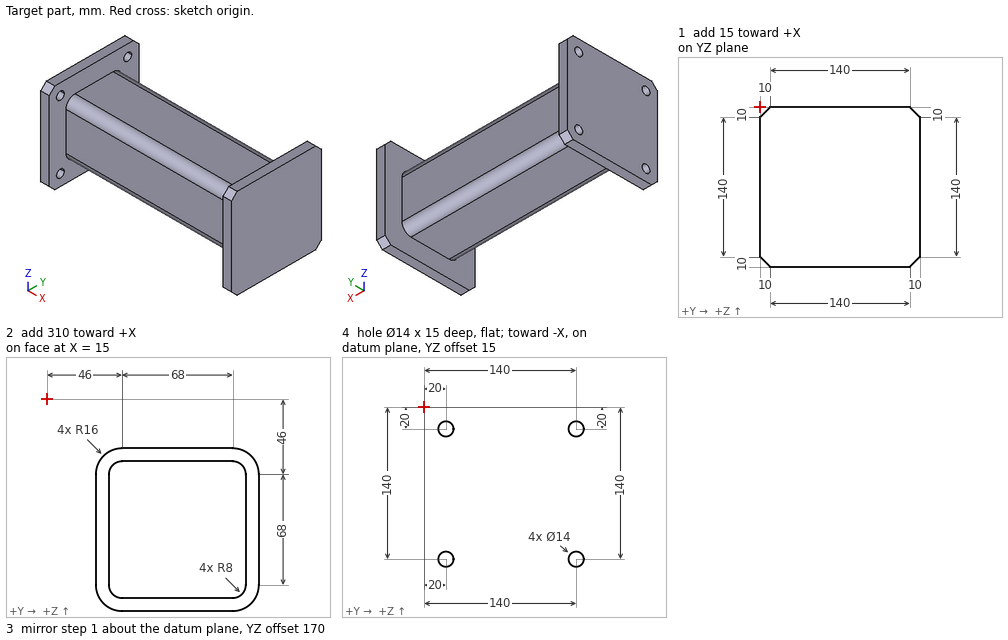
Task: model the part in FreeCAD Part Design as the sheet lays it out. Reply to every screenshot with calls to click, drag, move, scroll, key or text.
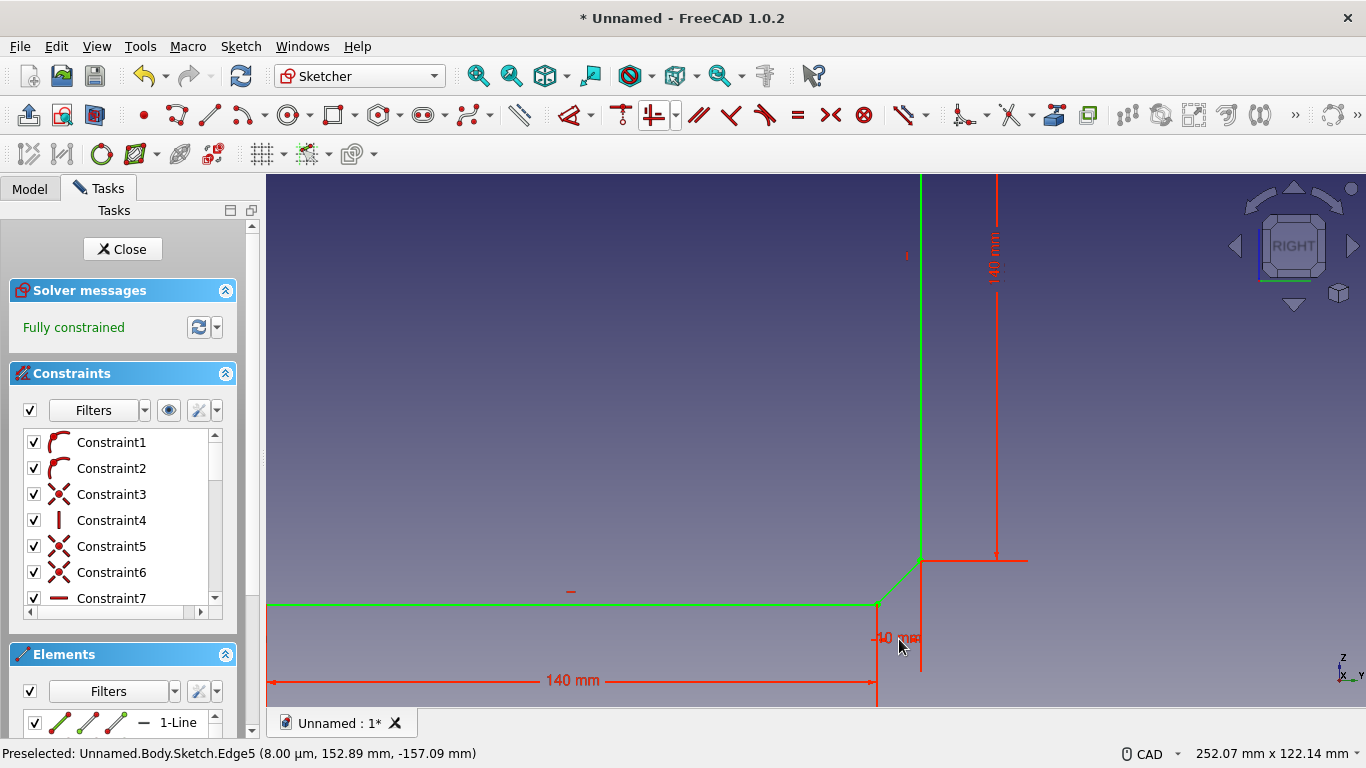
click(123, 249)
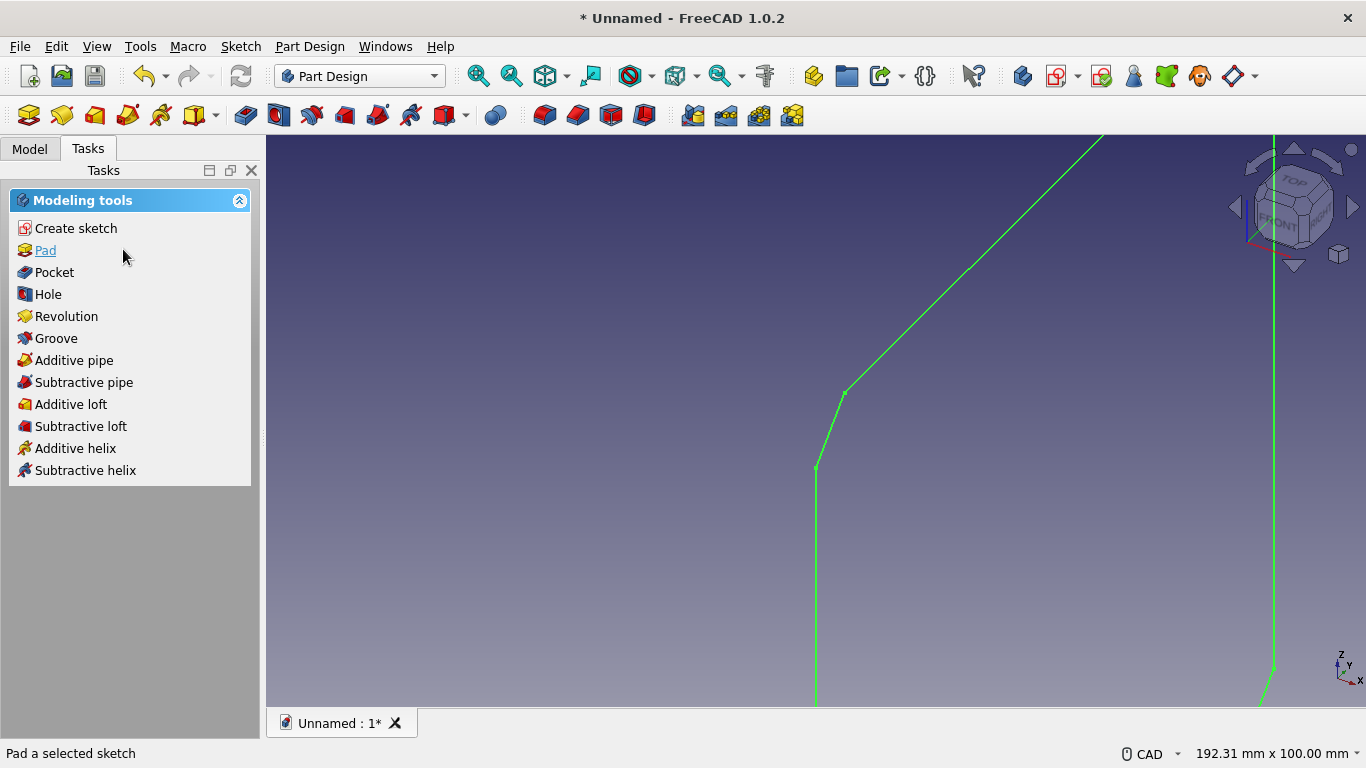
click(29, 116)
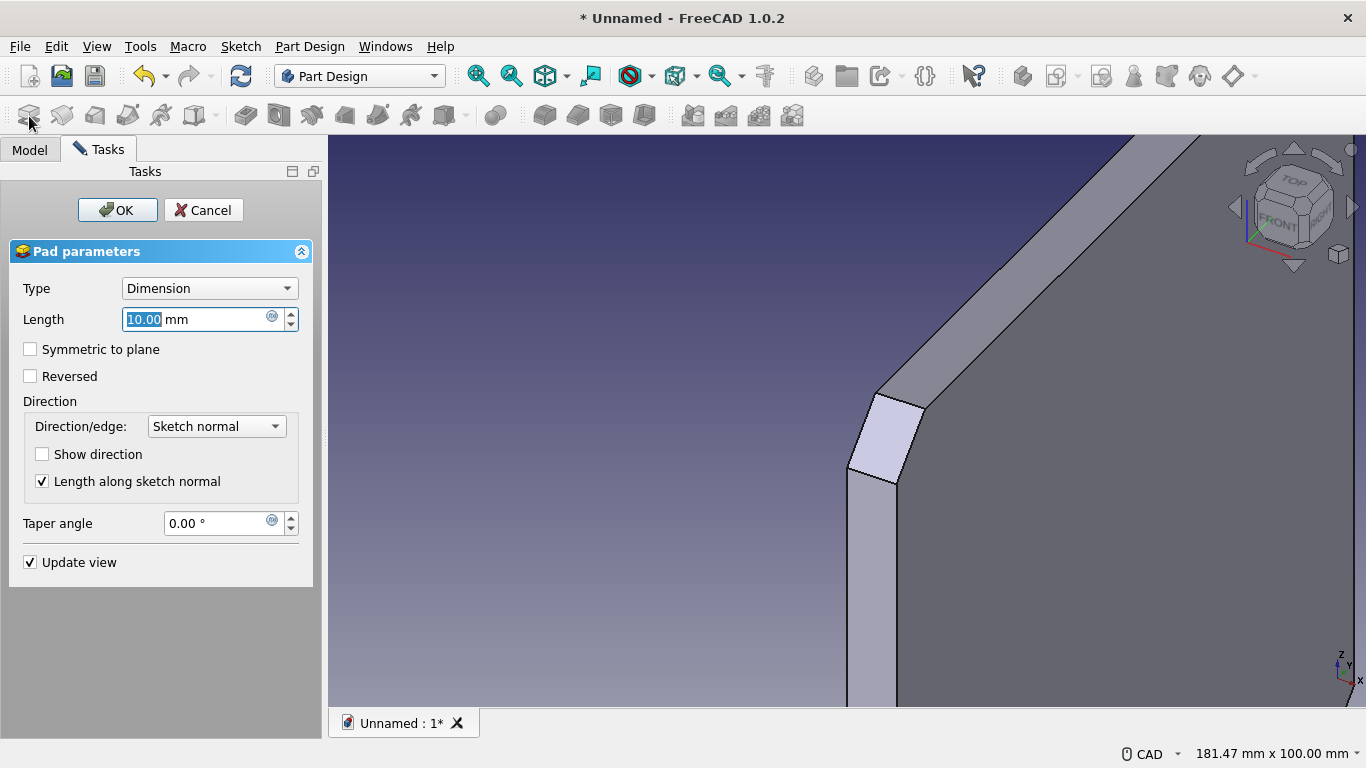
text(15)
key(Tab)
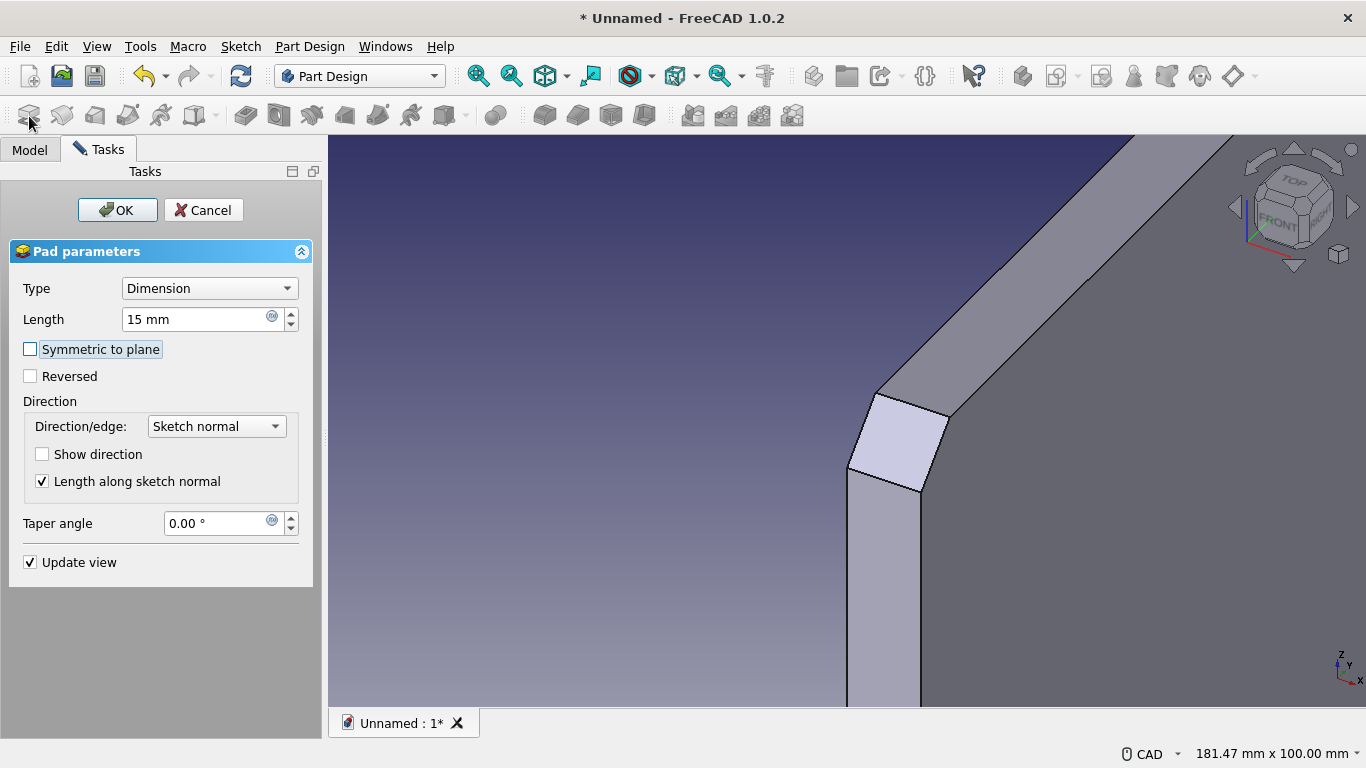
click(118, 210)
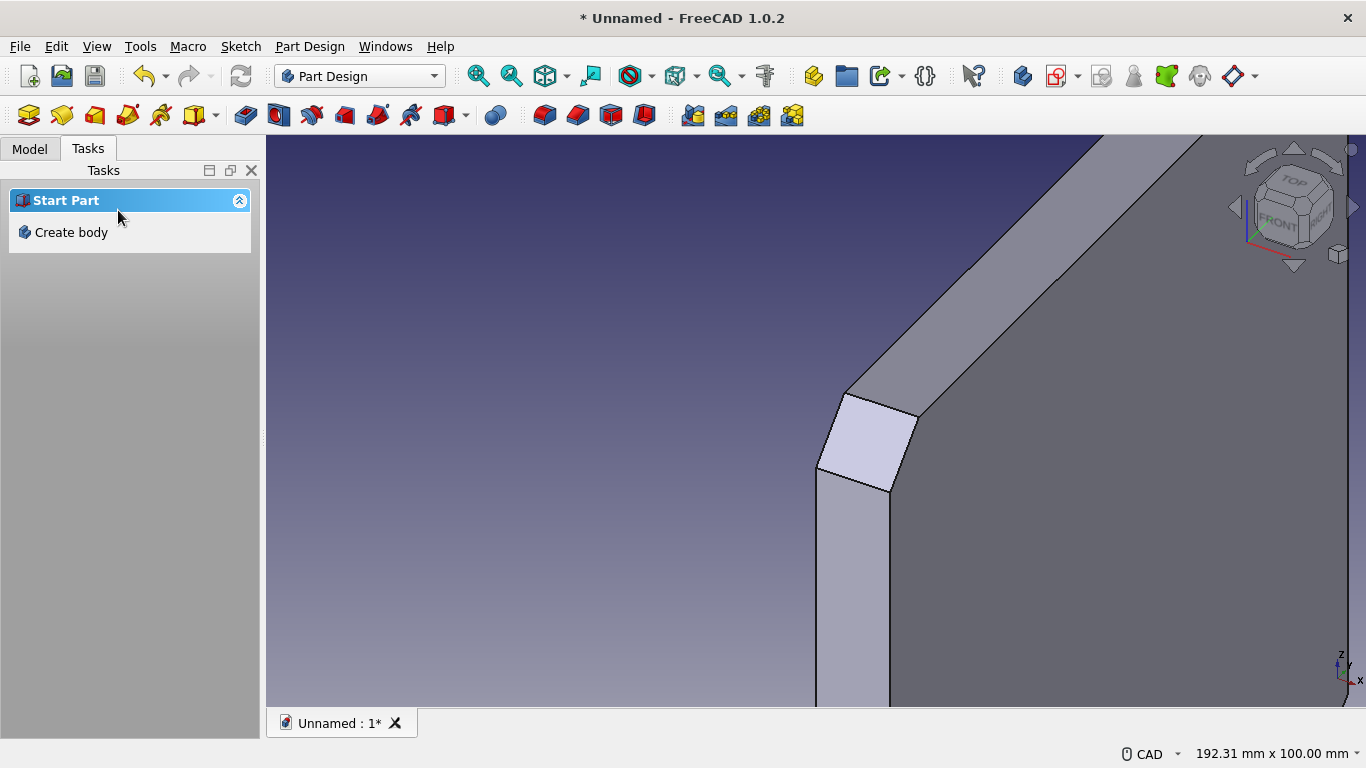
click(479, 76)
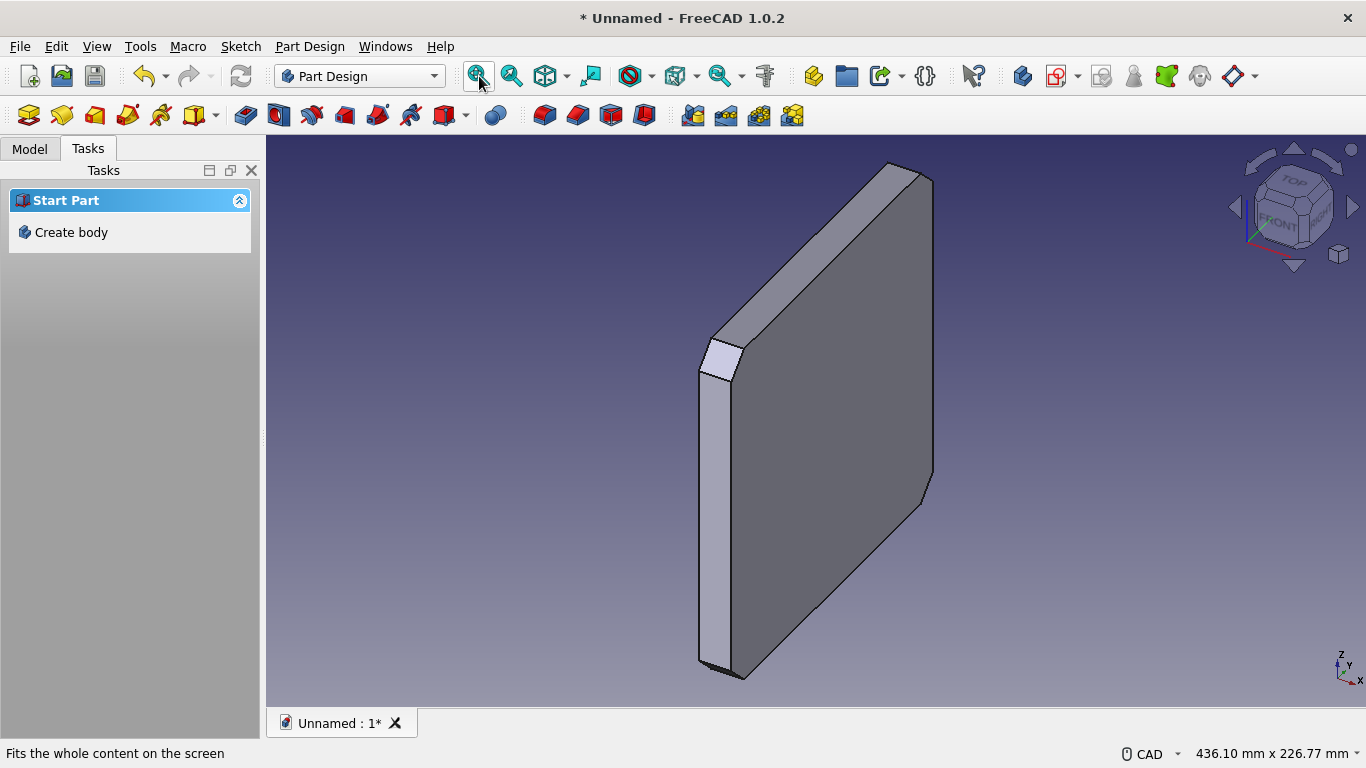
click(832, 425)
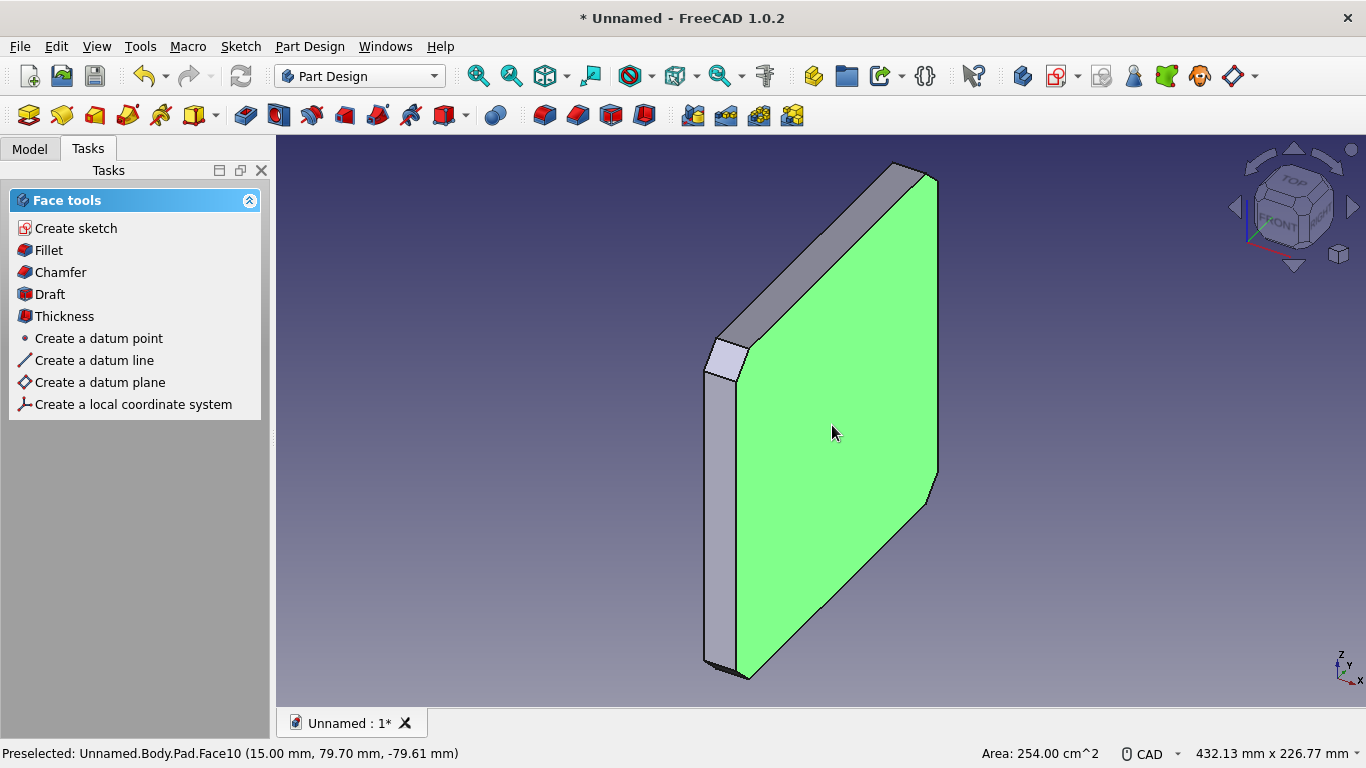
click(1056, 76)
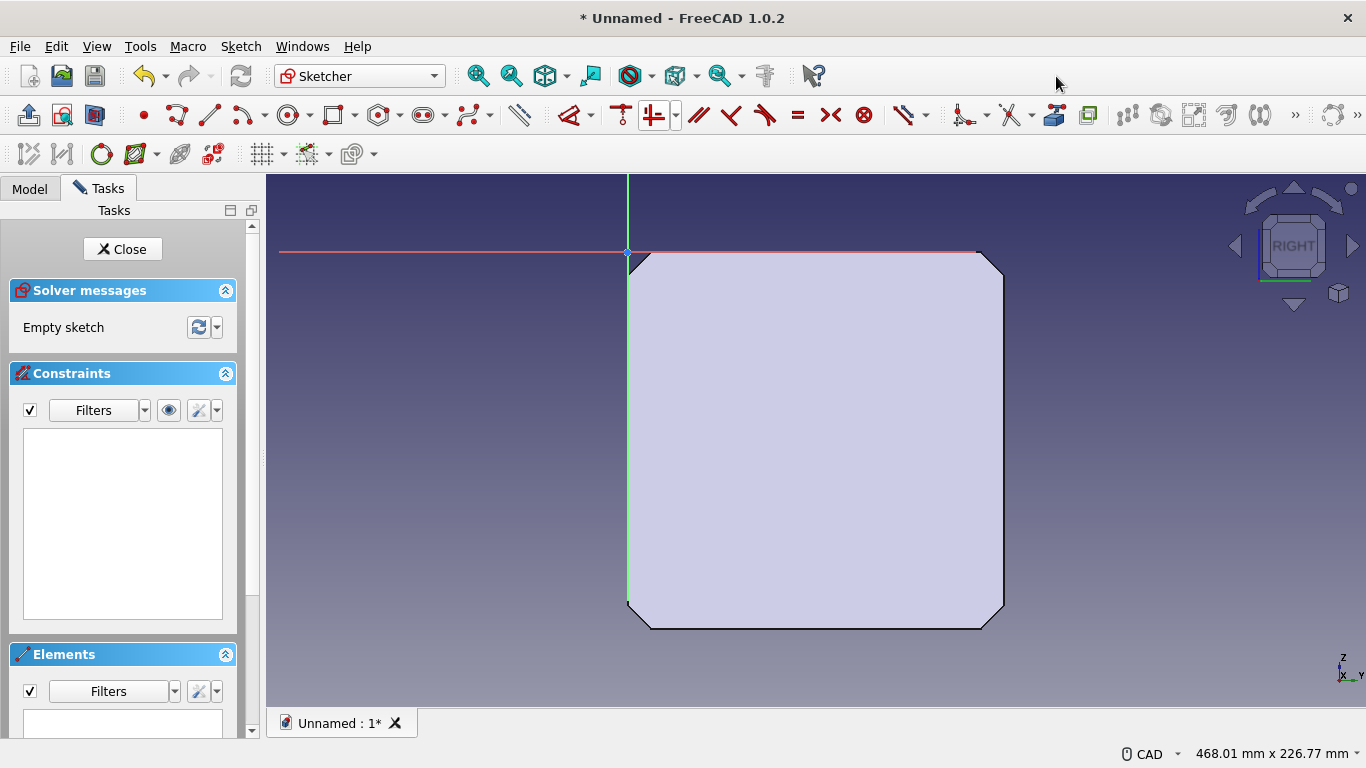
click(210, 116)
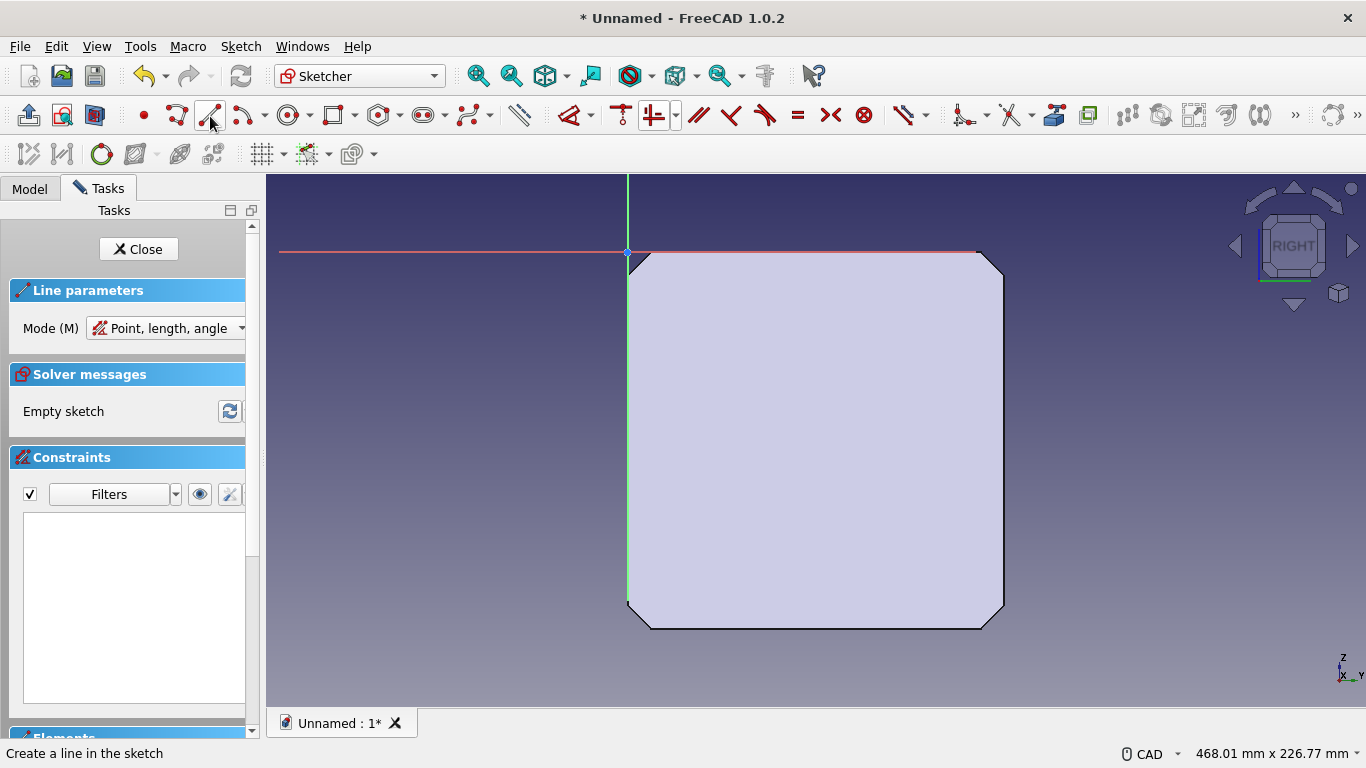
click(934, 520)
click(934, 361)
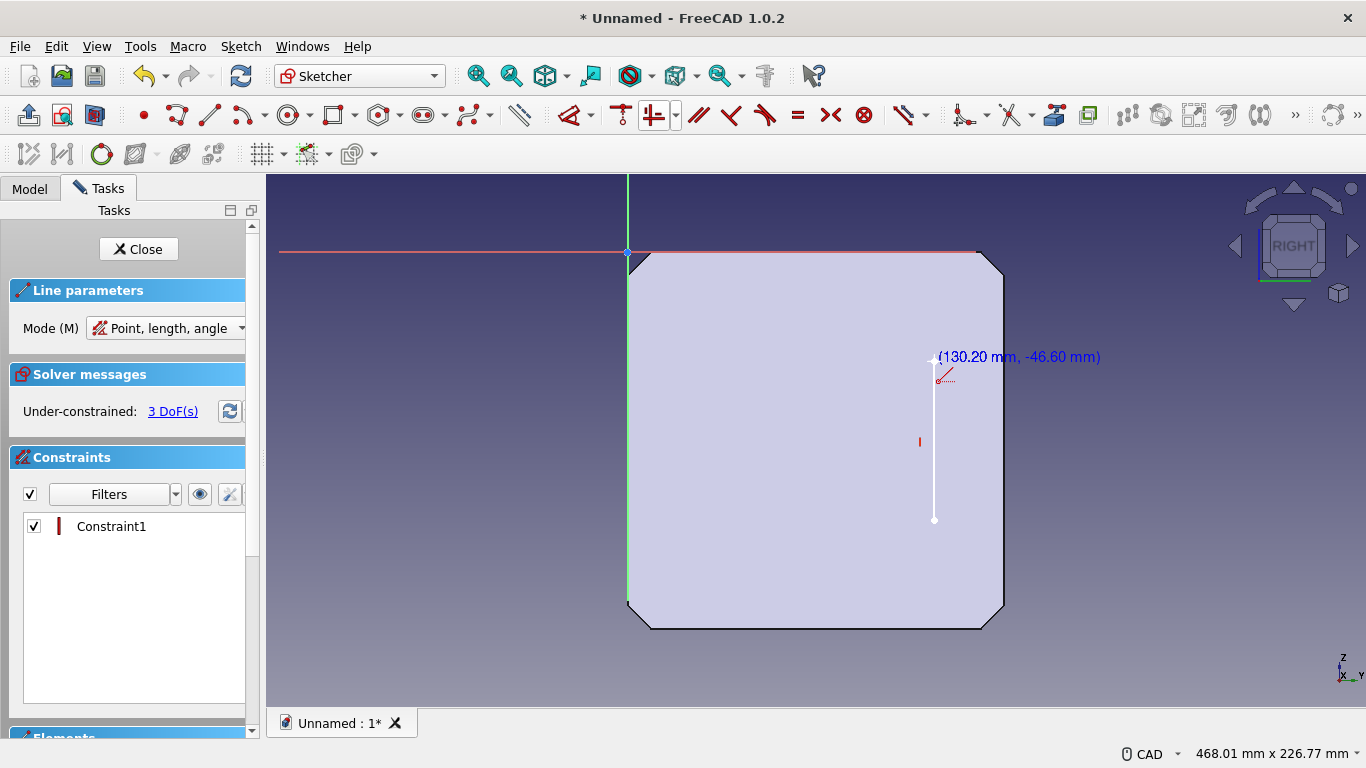
click(896, 323)
click(736, 323)